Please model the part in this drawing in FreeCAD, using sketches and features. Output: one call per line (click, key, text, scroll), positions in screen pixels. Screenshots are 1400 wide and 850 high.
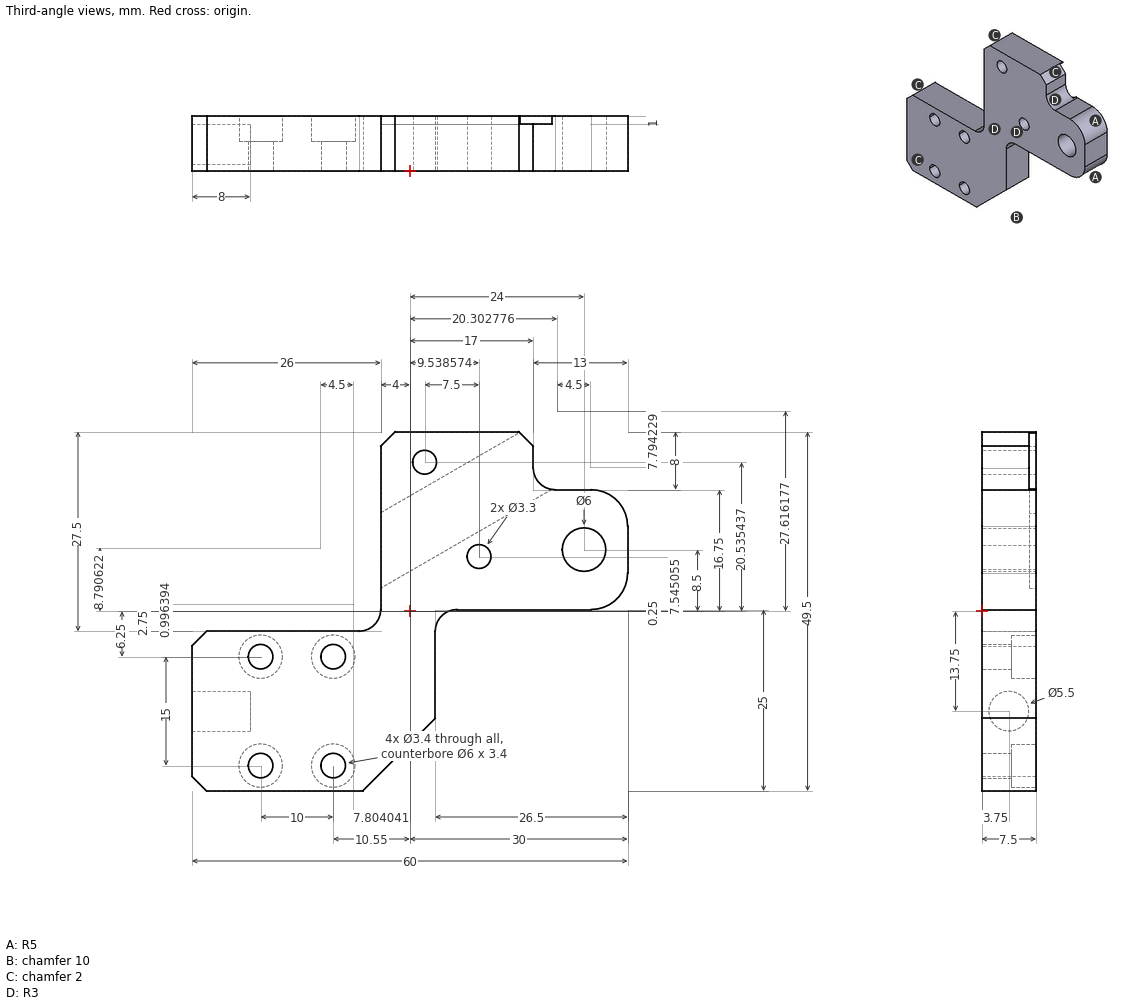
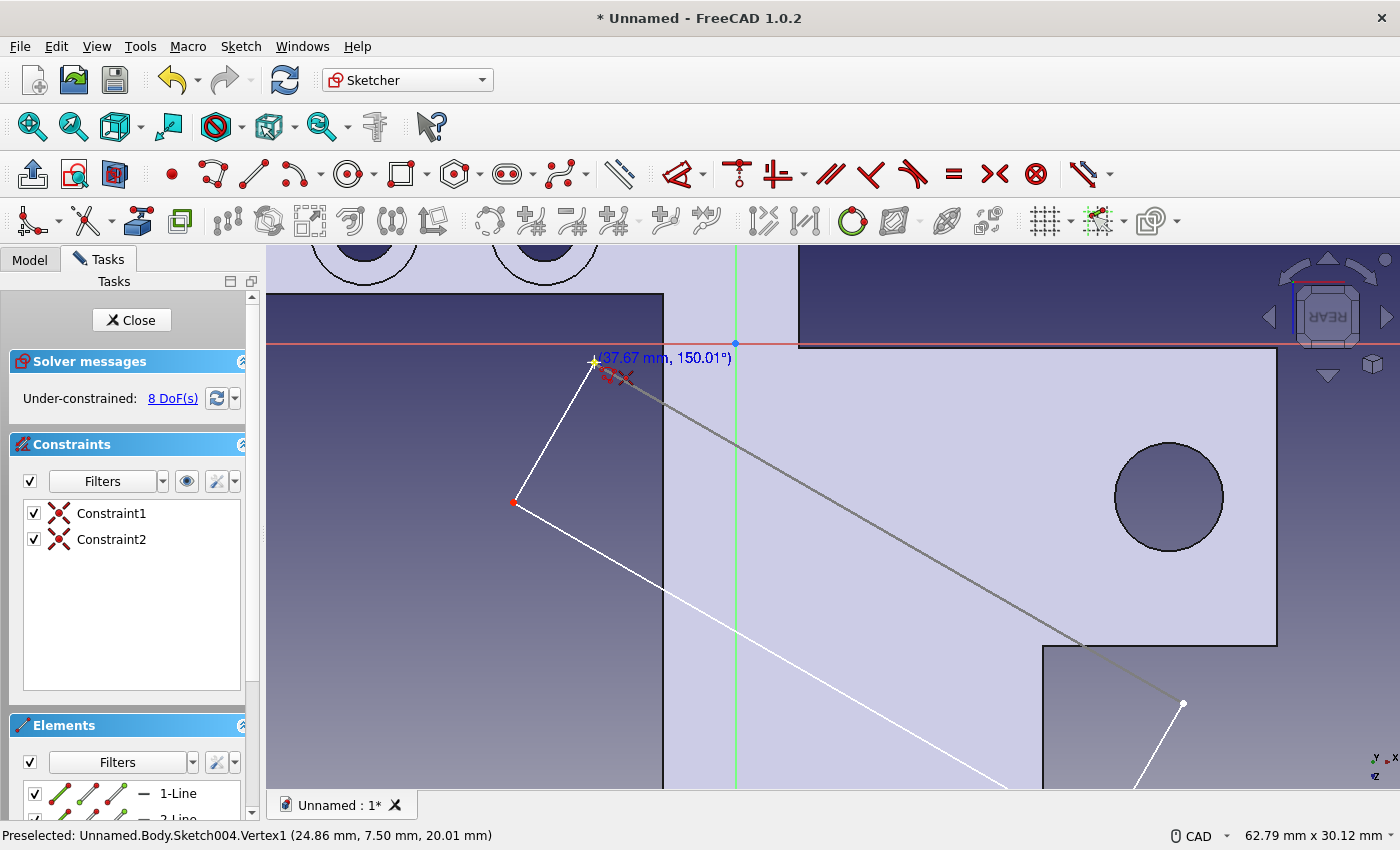
click(594, 363)
key(Escape)
key(Escape)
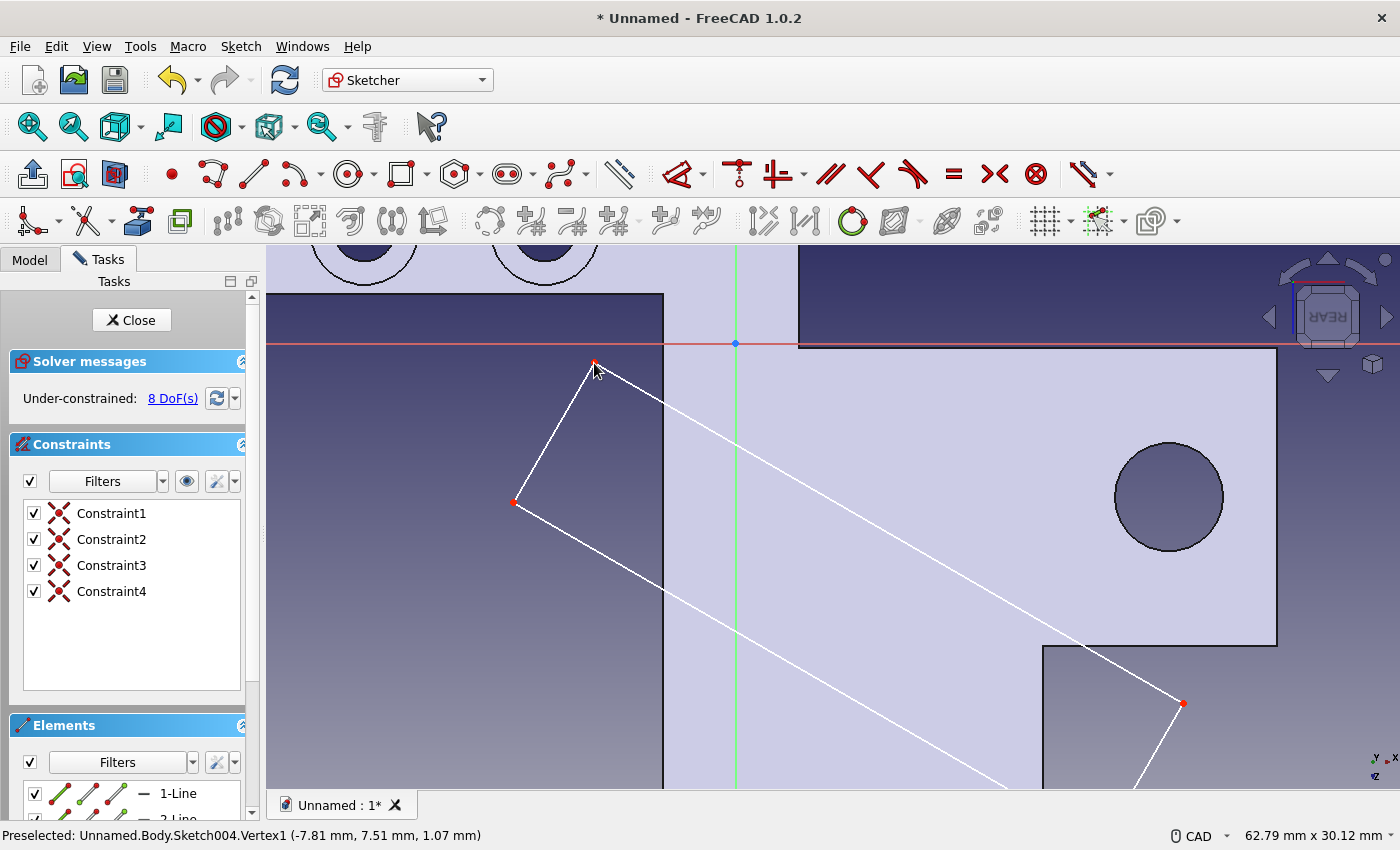
key(d)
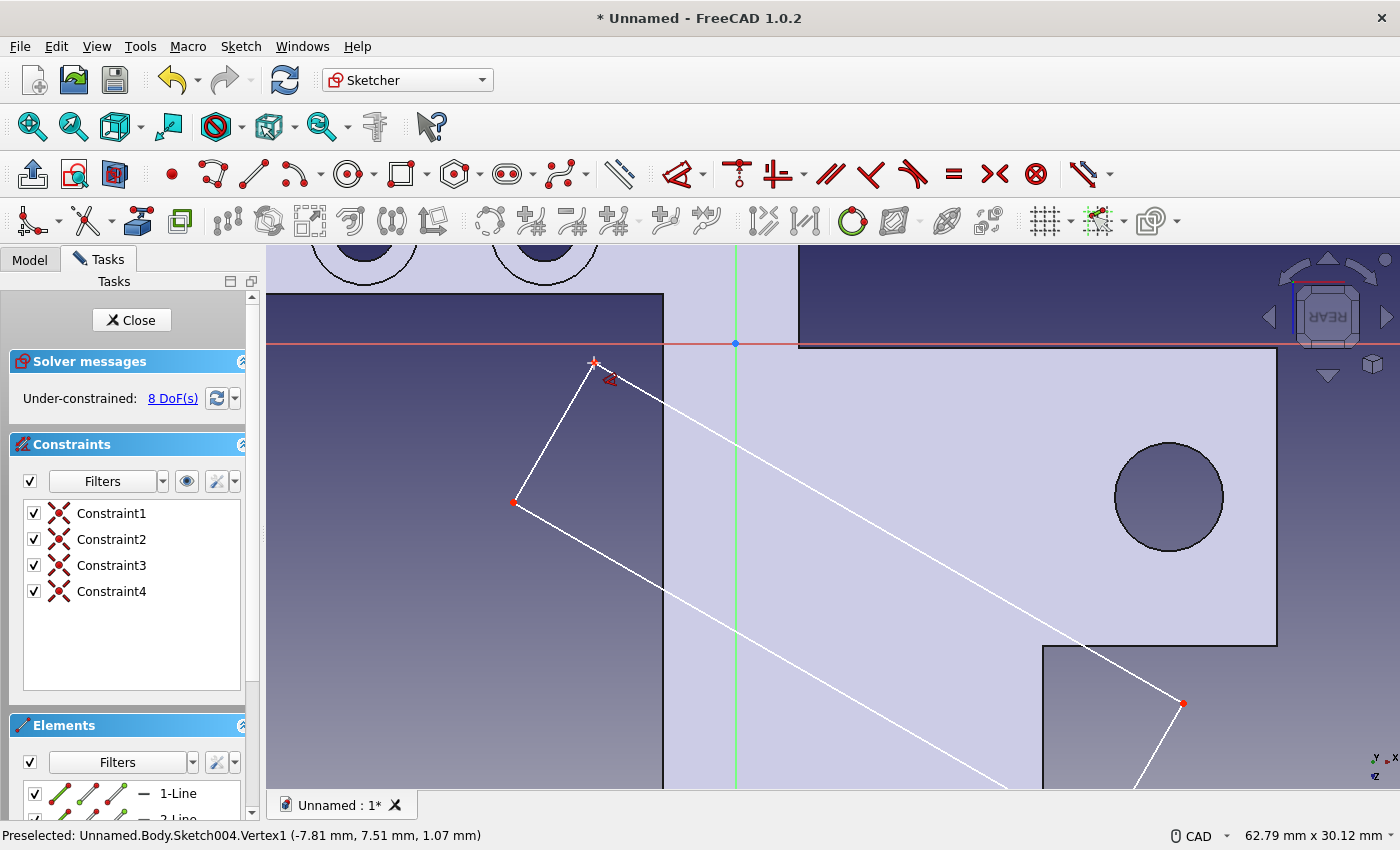
click(570, 405)
click(554, 329)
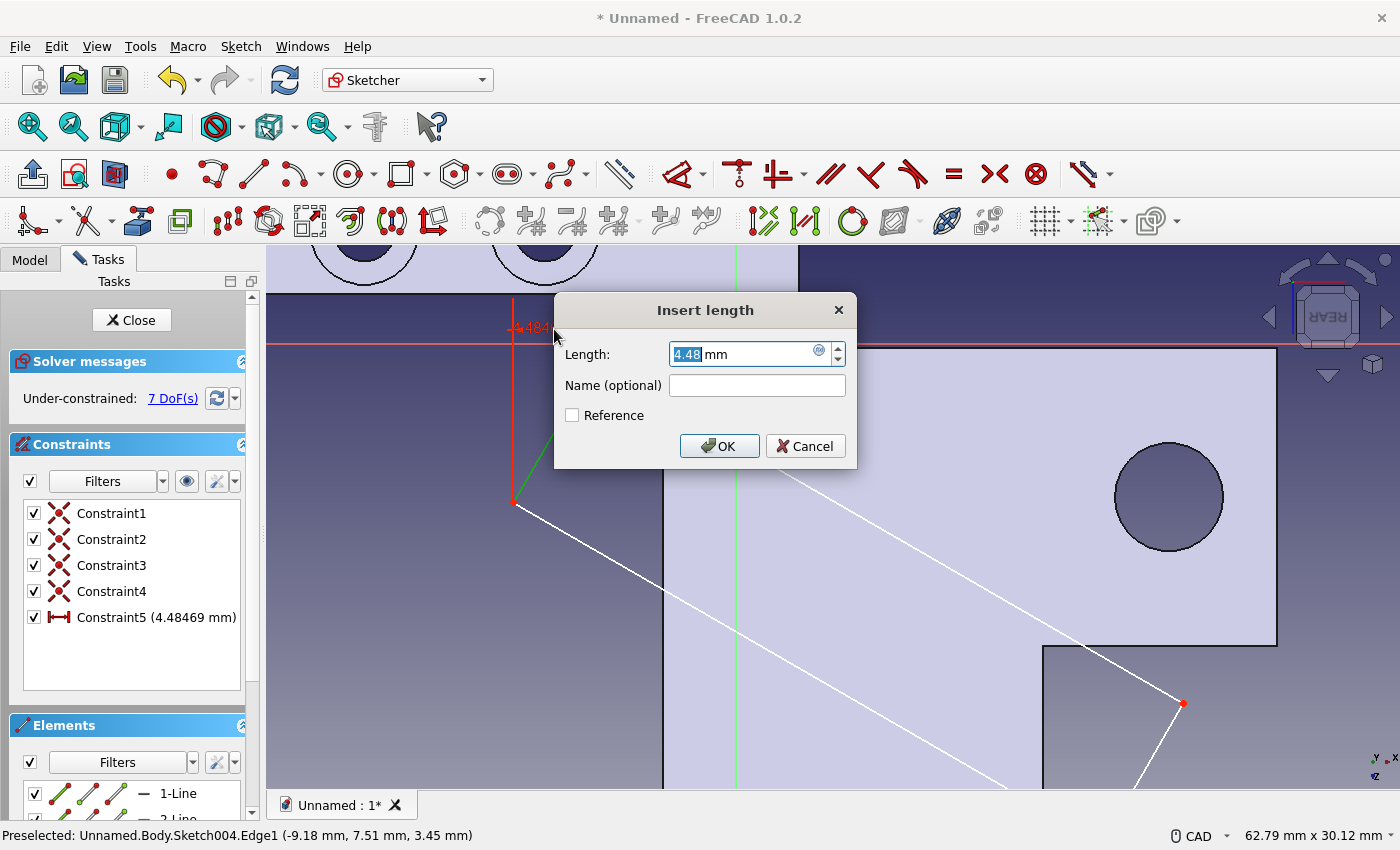
text(4.5)
key(Return)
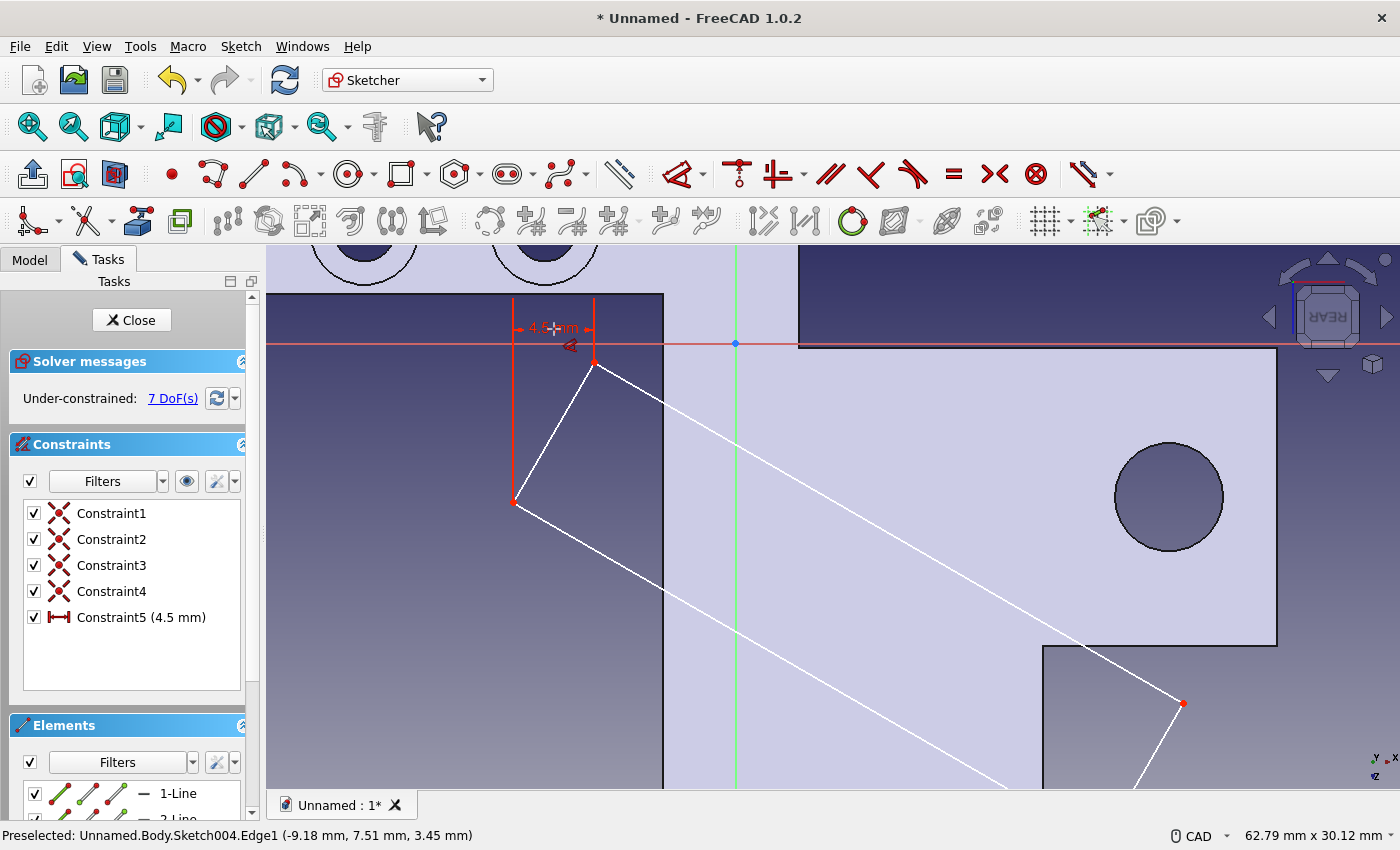
click(1159, 746)
click(1161, 670)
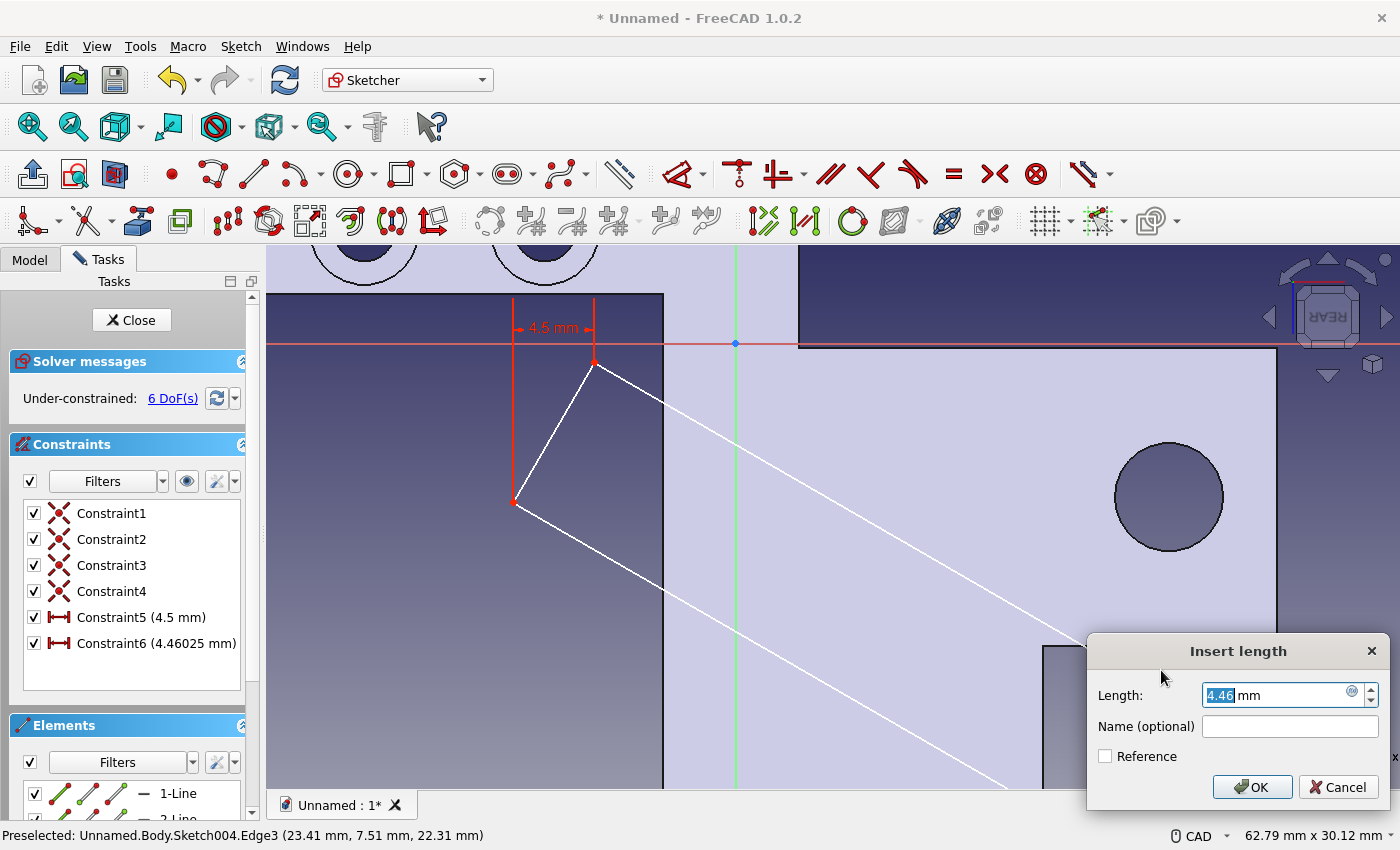
text(4.5)
key(Return)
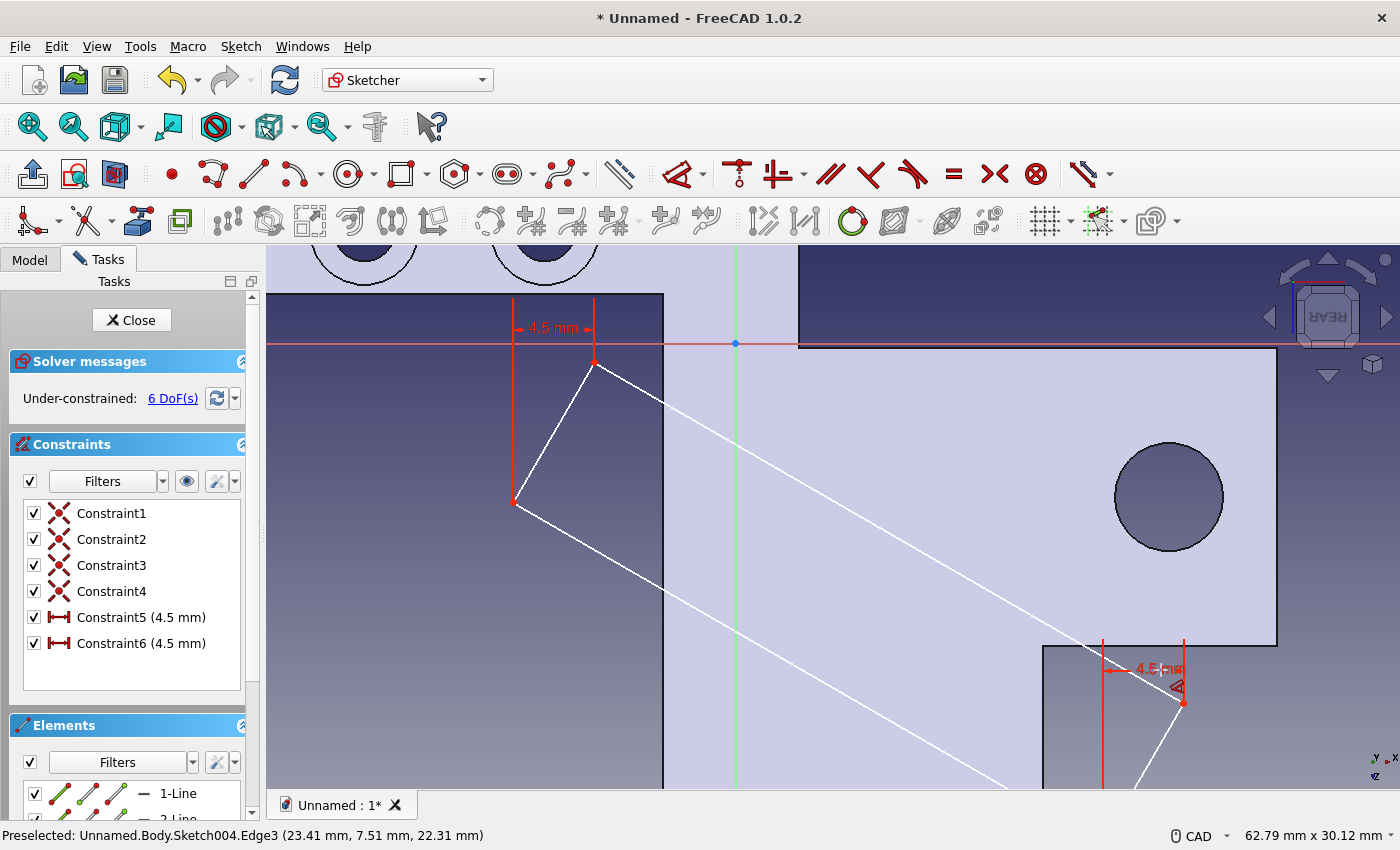
click(594, 363)
click(665, 310)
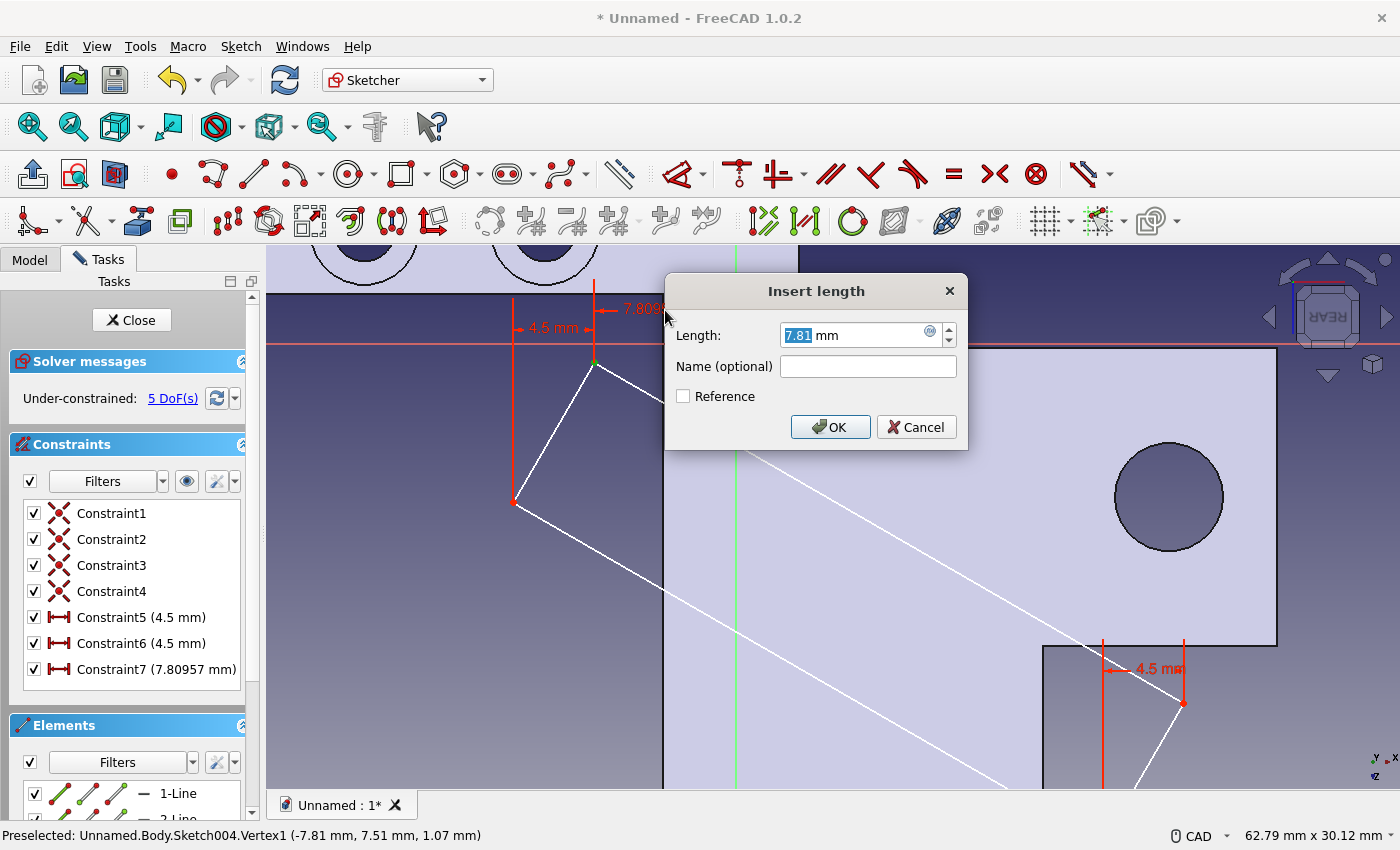
text(7.804041)
key(Return)